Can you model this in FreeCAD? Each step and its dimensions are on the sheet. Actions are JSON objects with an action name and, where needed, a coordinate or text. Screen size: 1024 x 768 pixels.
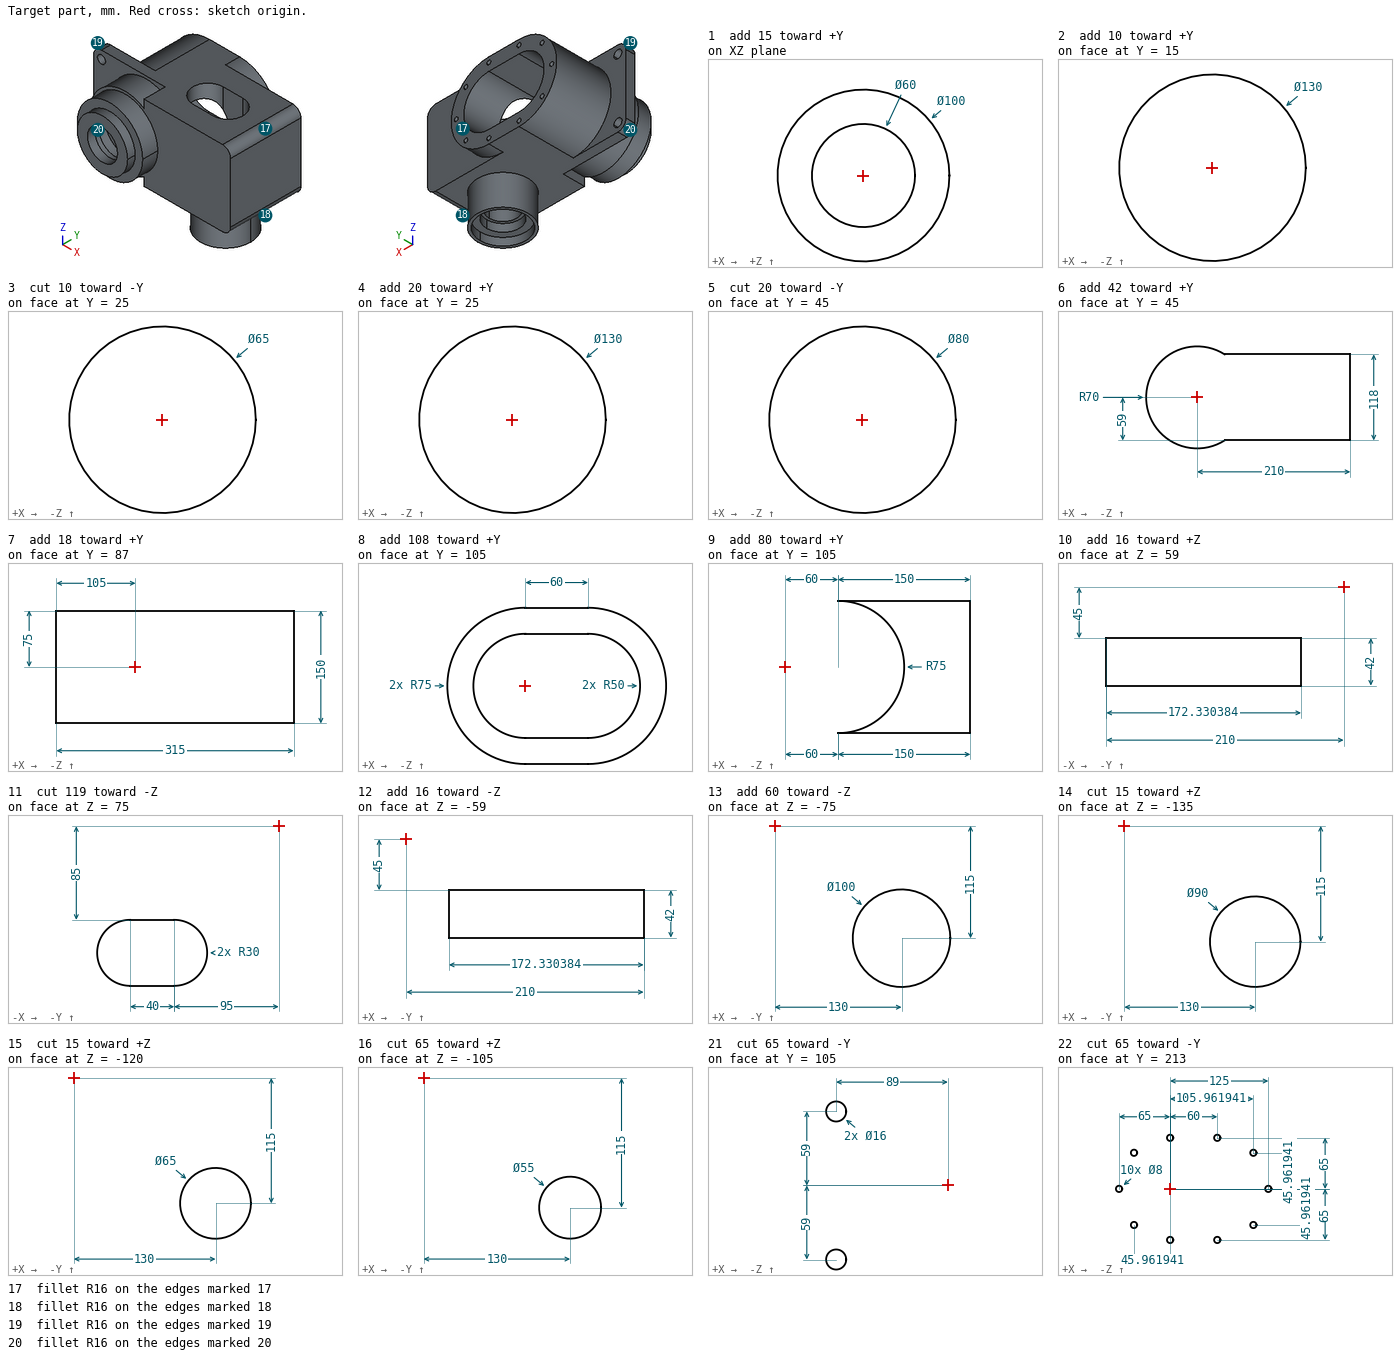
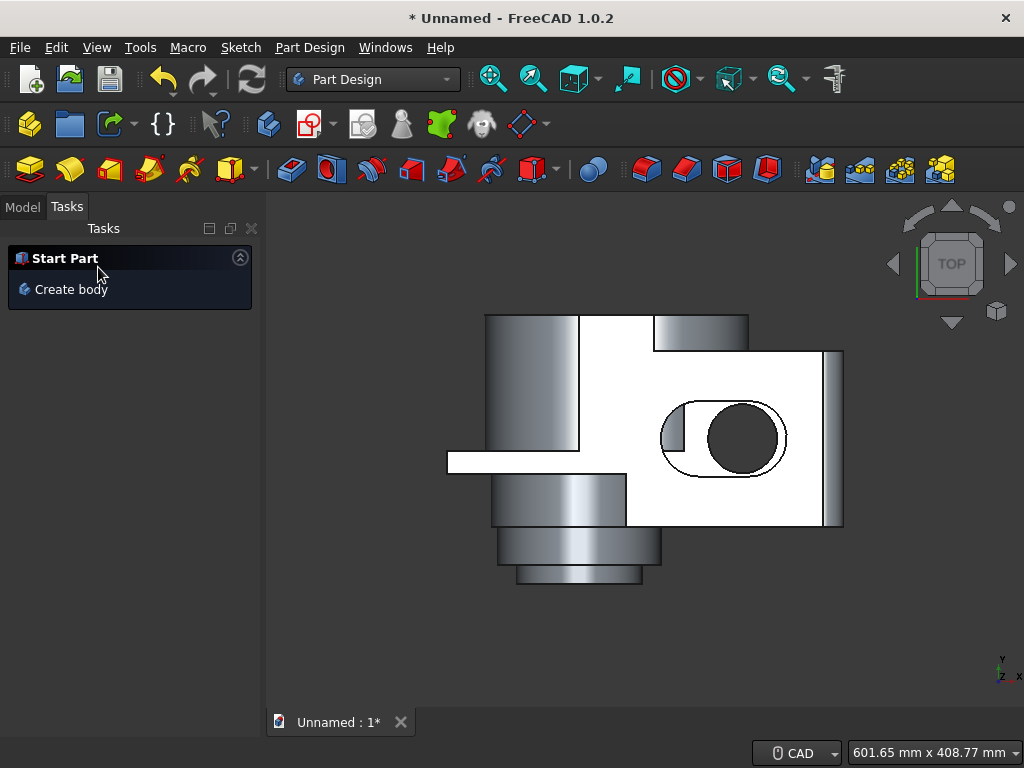
{"action": "key", "text": "0"}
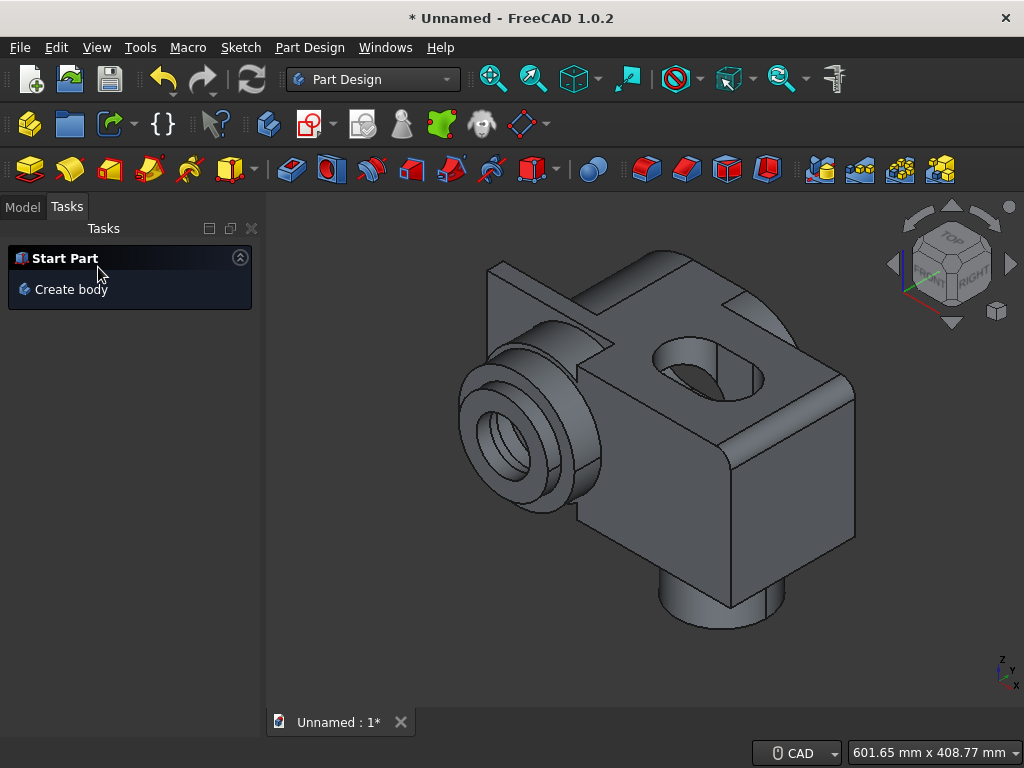
{"action": "key", "text": "1"}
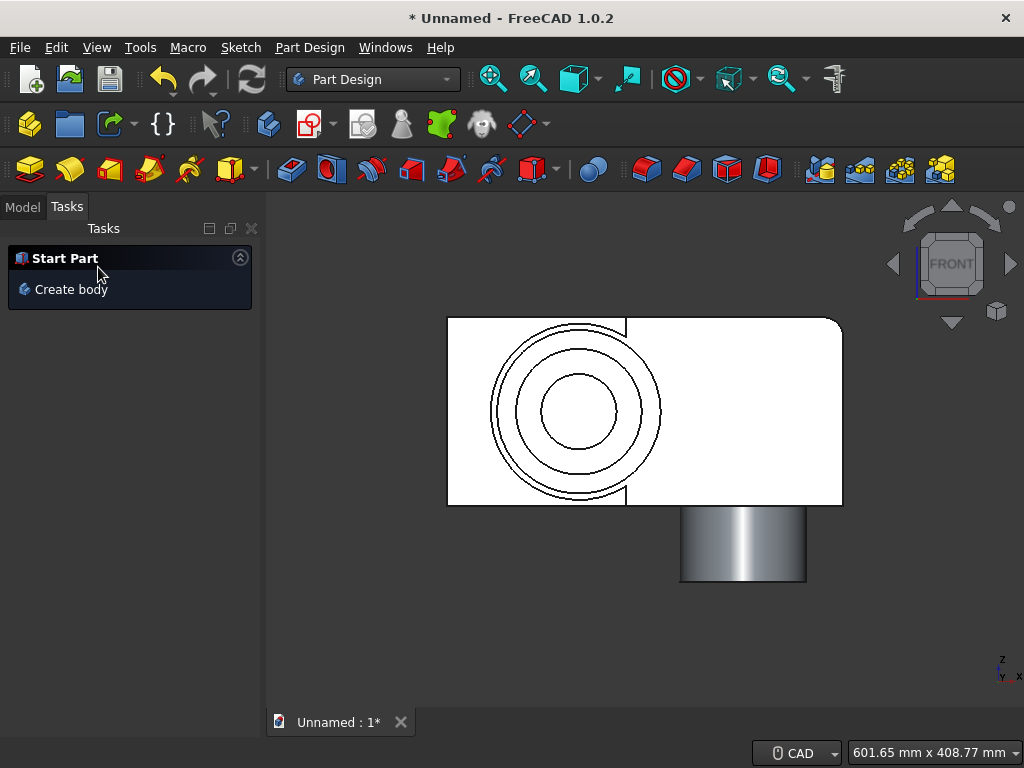
{"action": "key", "text": "3"}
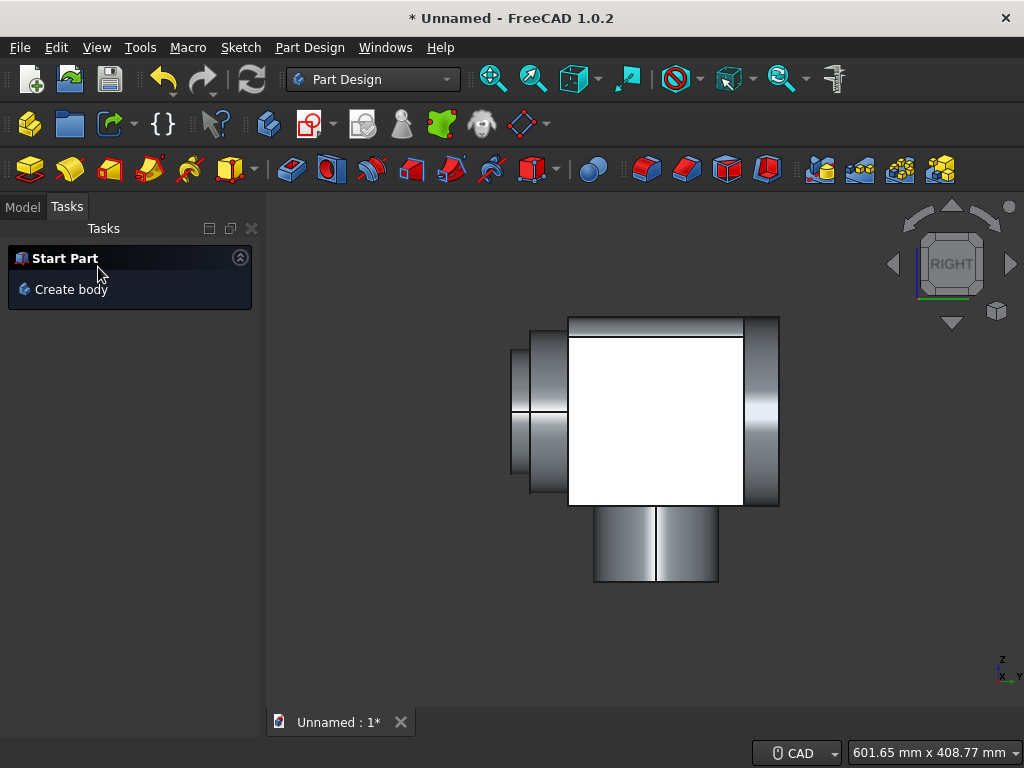
{"action": "left_click", "coordinate": [656, 505]}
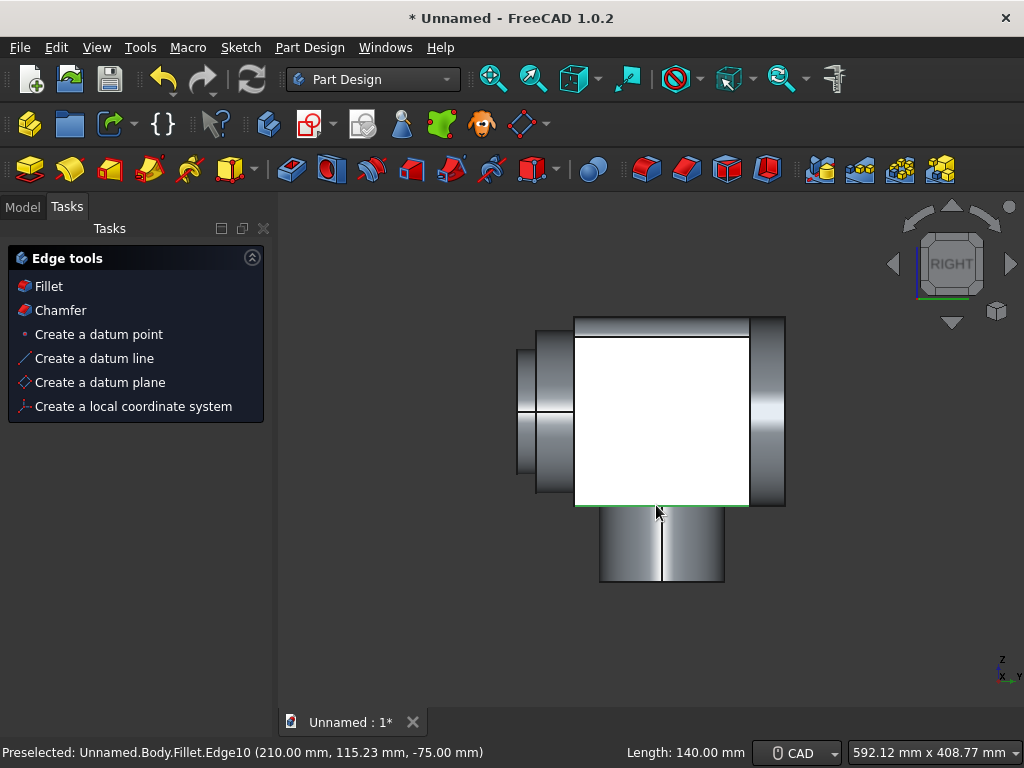
{"action": "left_click", "coordinate": [648, 170]}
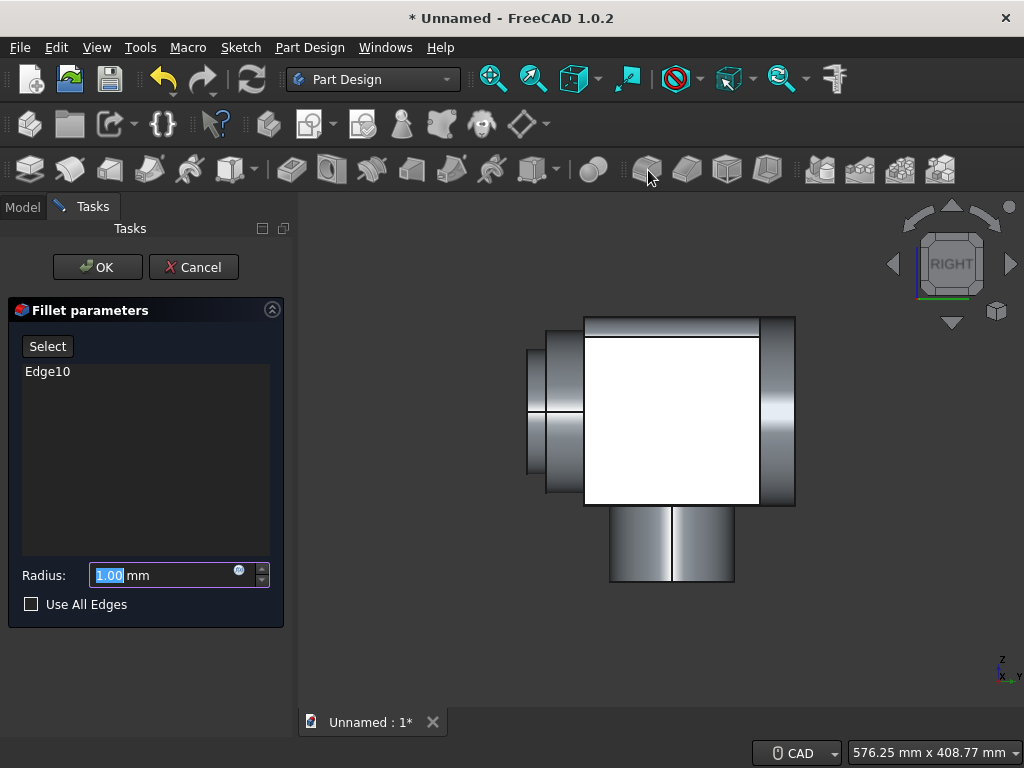
{"action": "type", "text": "16"}
{"action": "key", "text": "Tab"}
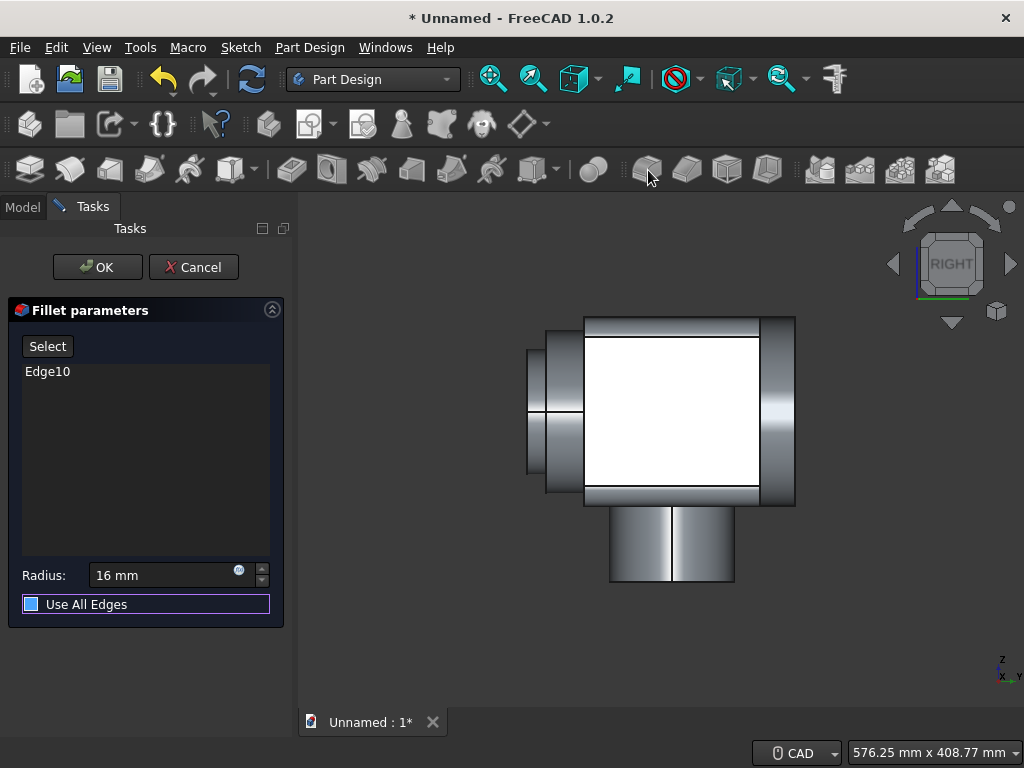
{"action": "left_click", "coordinate": [98, 267]}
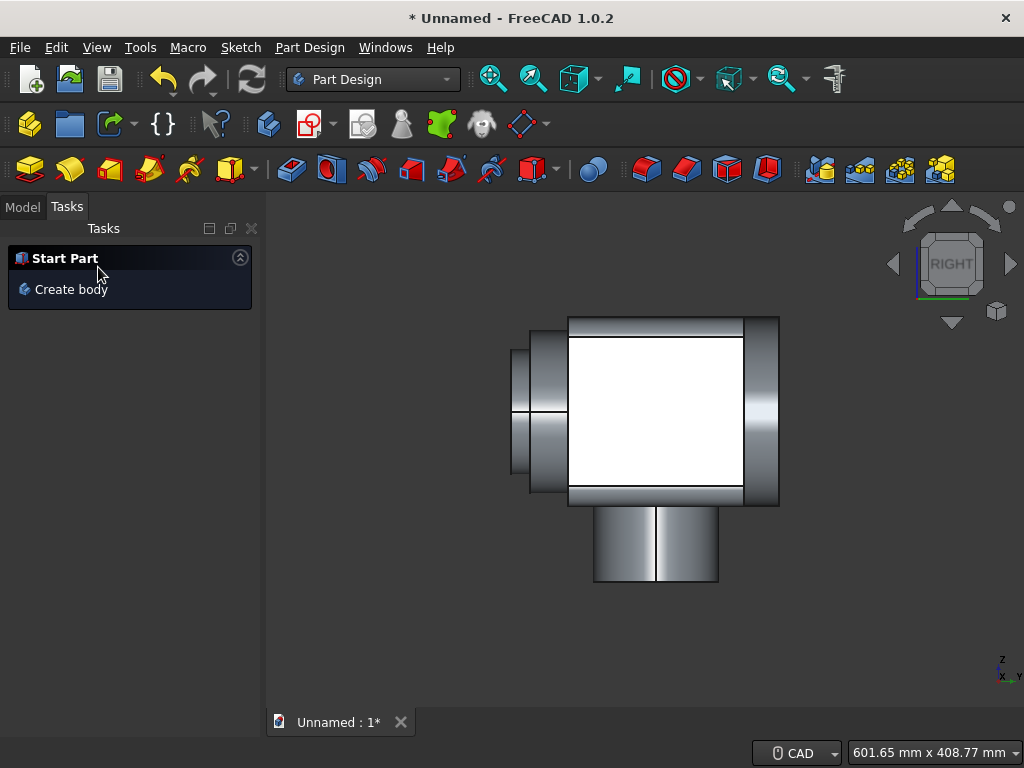
{"action": "key", "text": "0"}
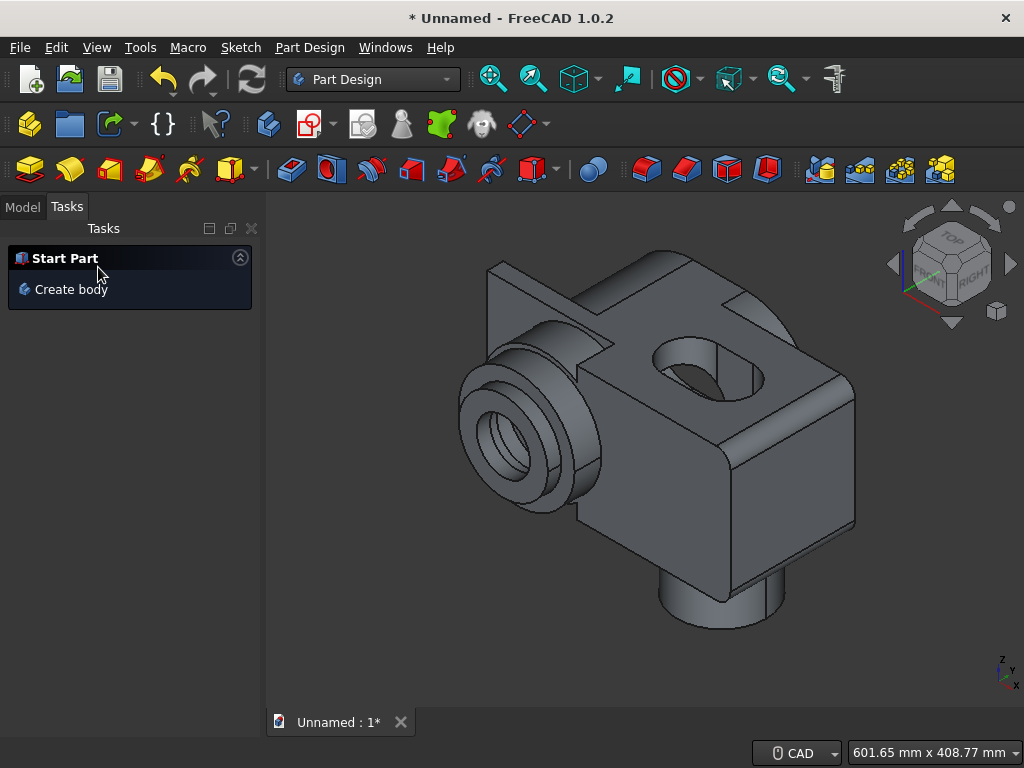
{"action": "key", "text": "2"}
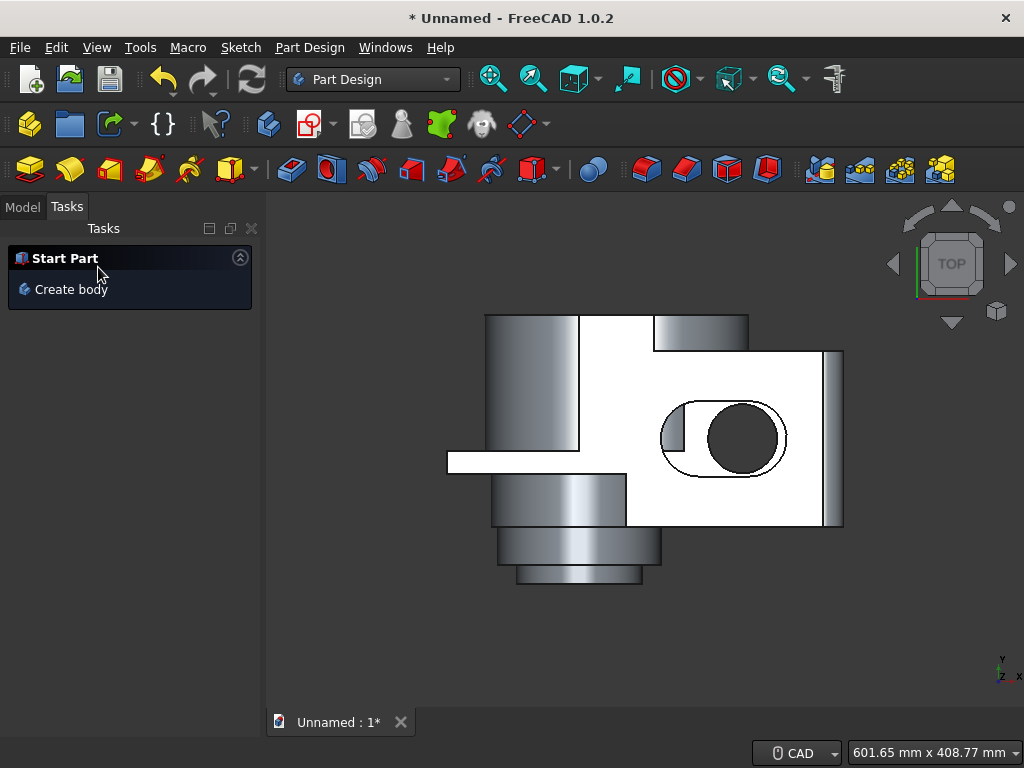
{"action": "left_click", "coordinate": [447, 462]}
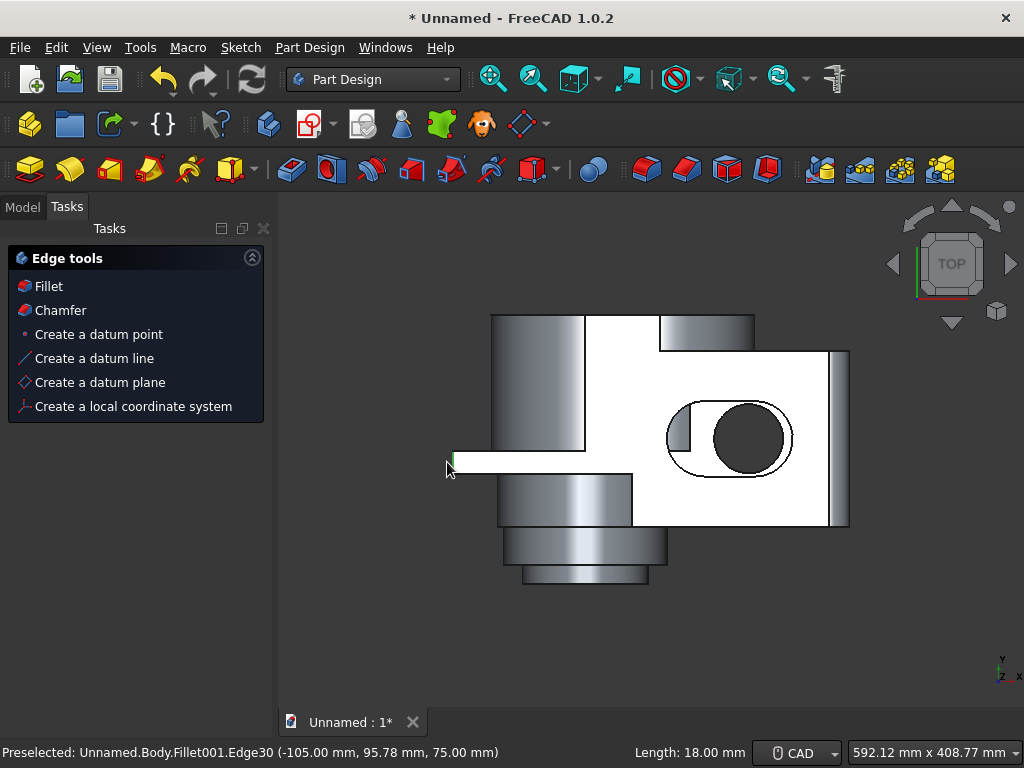
{"action": "left_click", "coordinate": [648, 170]}